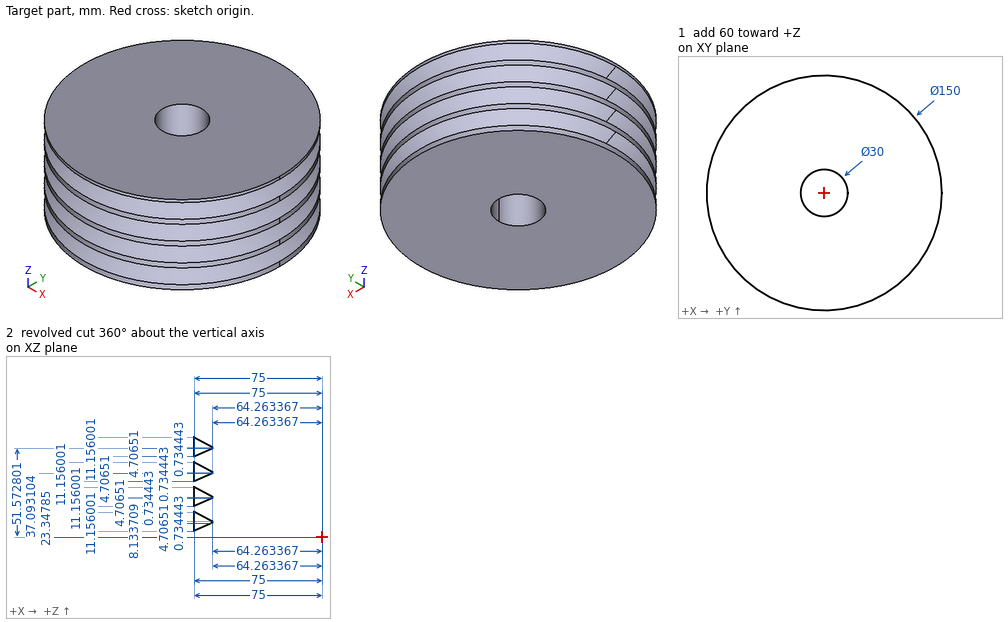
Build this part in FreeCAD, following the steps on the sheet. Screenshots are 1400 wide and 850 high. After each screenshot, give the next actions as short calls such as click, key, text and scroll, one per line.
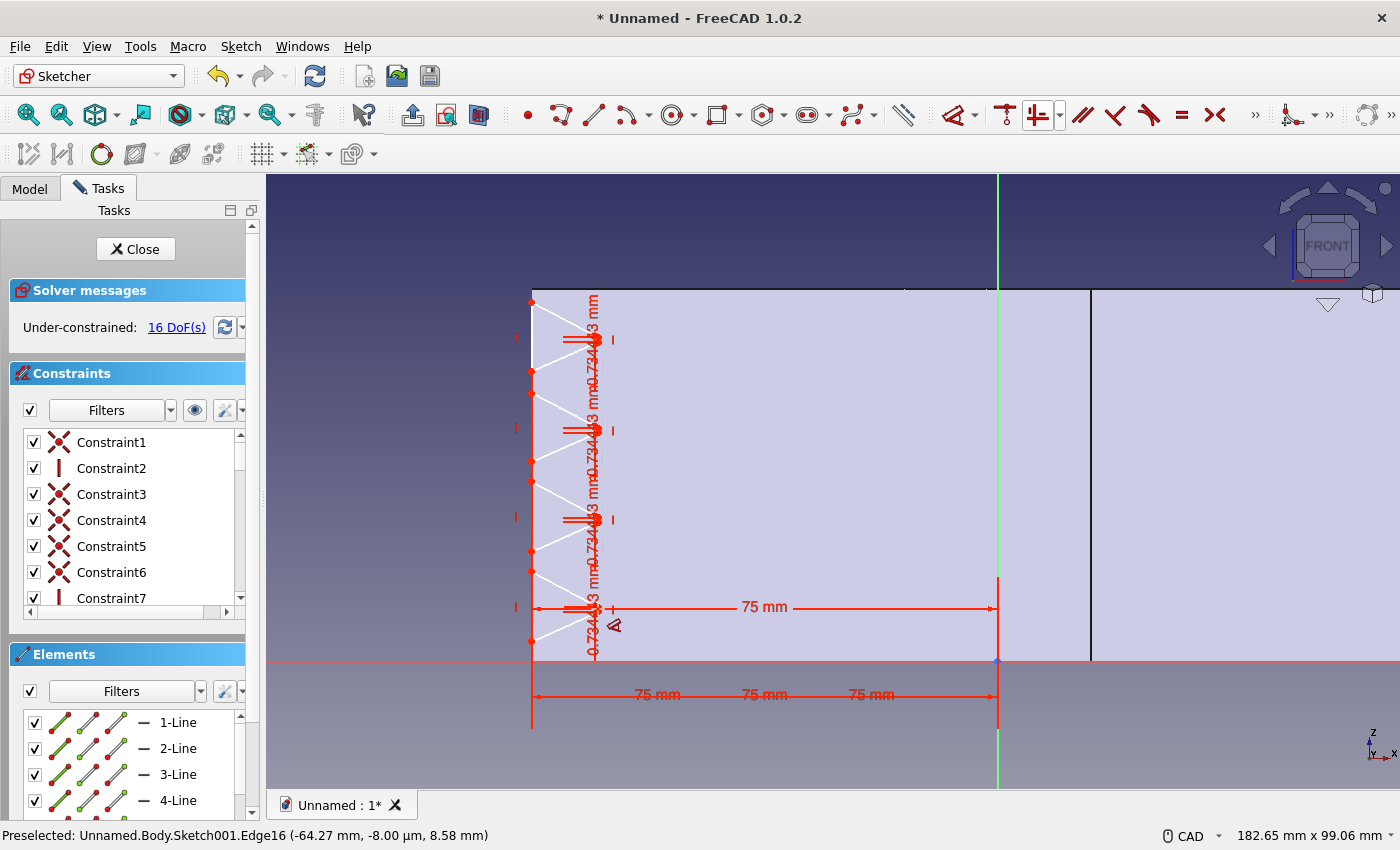
scroll(578, 351, up, 2)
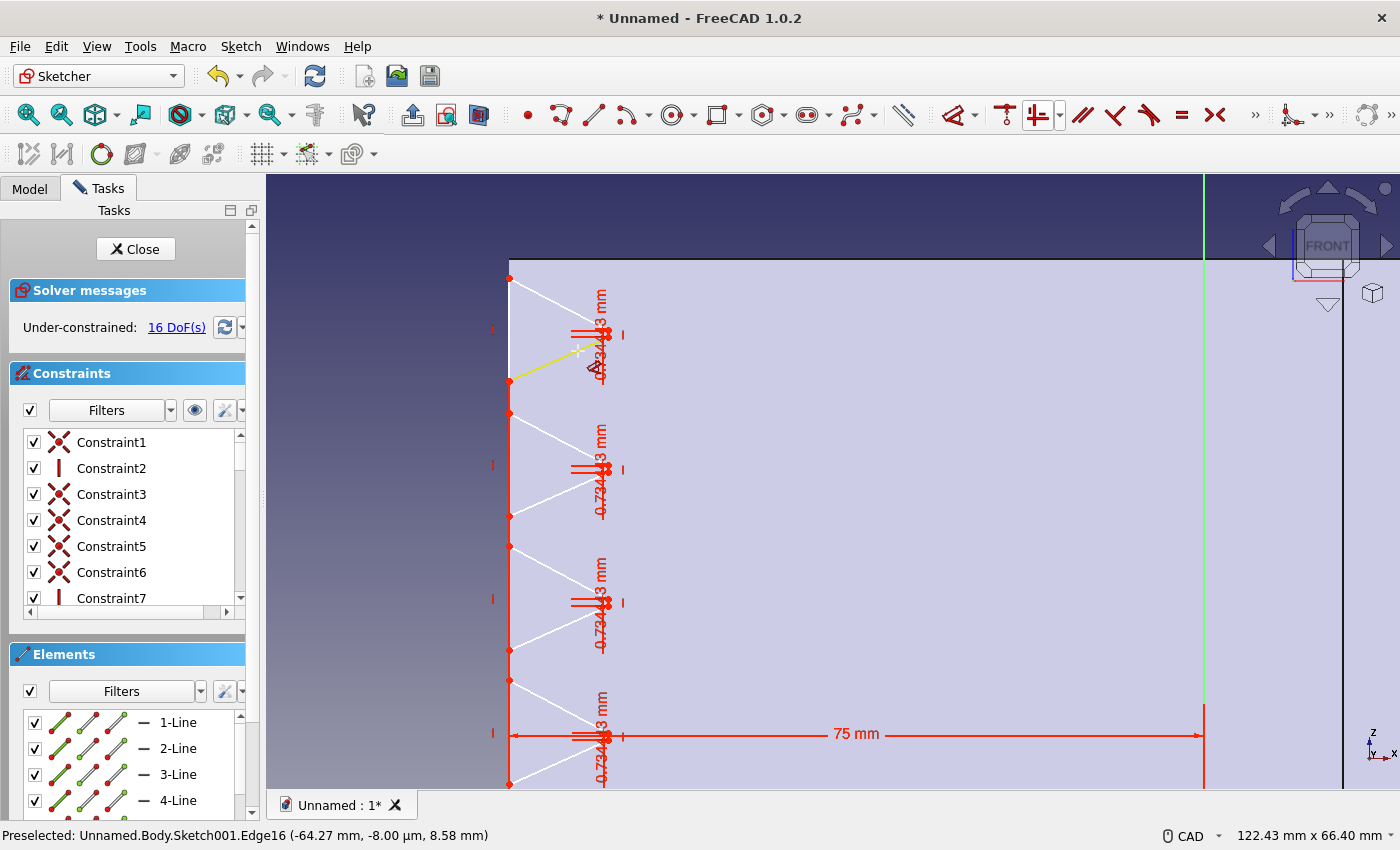
click(579, 351)
click(475, 359)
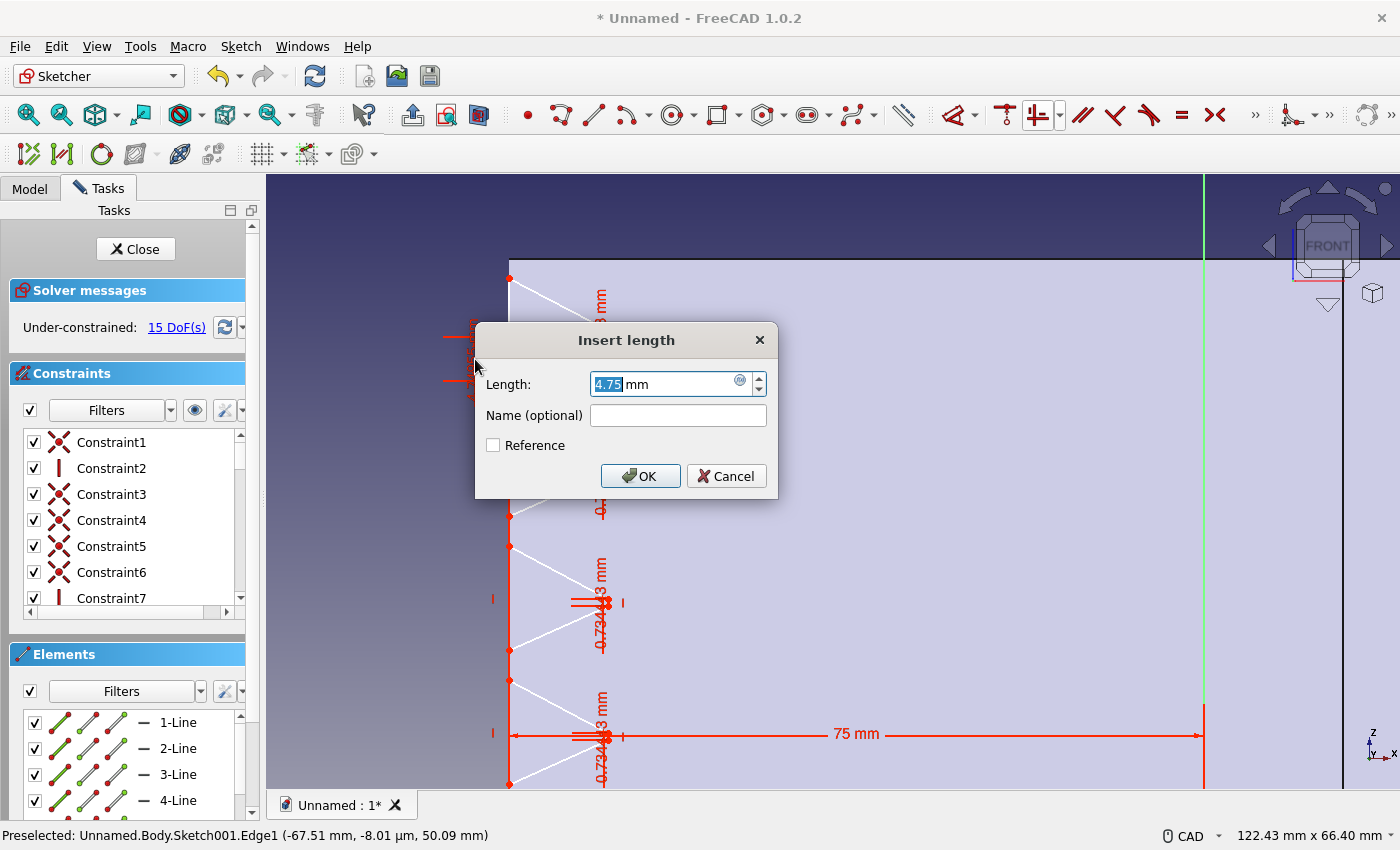
text(4.70651)
key(Return)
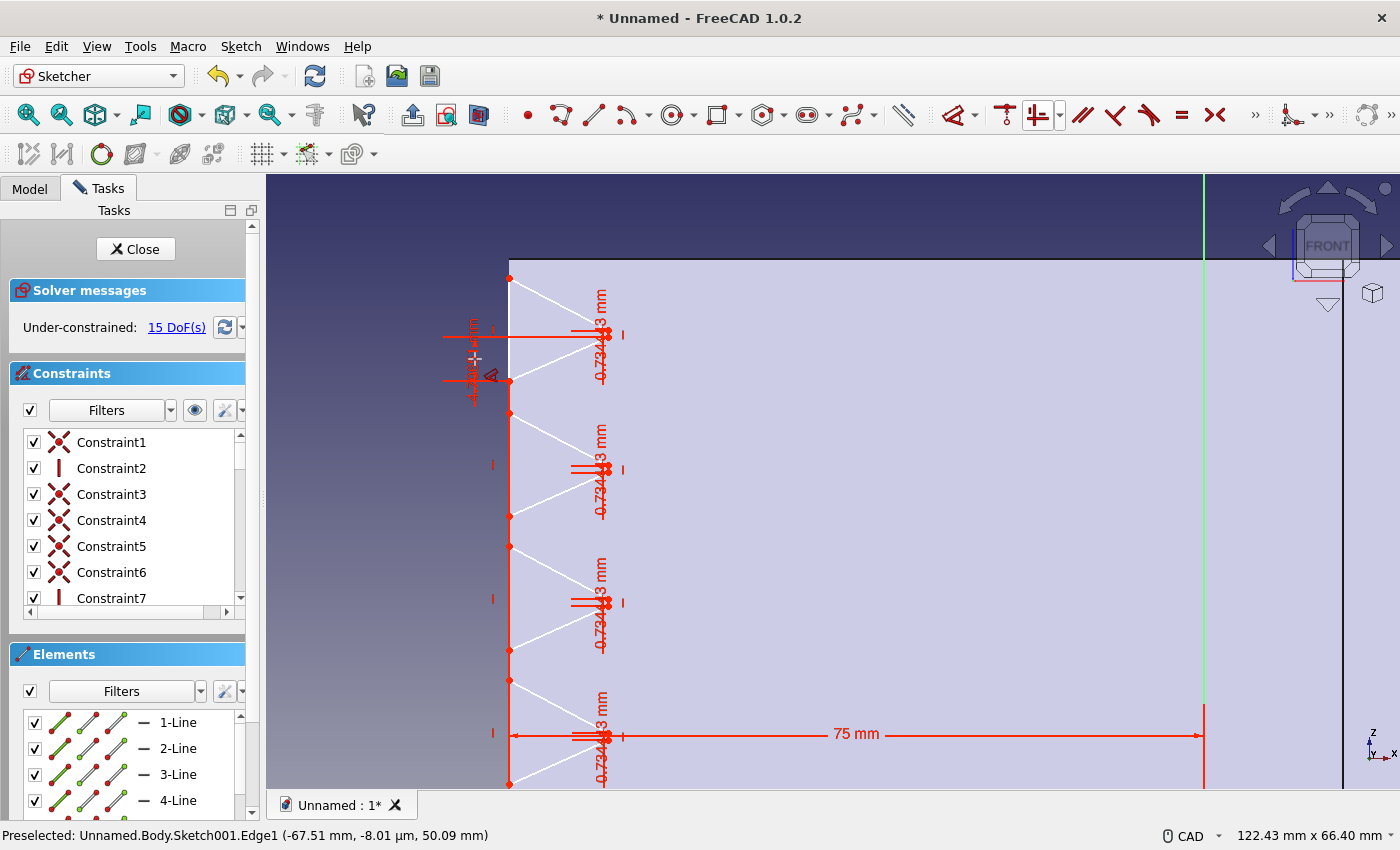
click(579, 486)
click(475, 494)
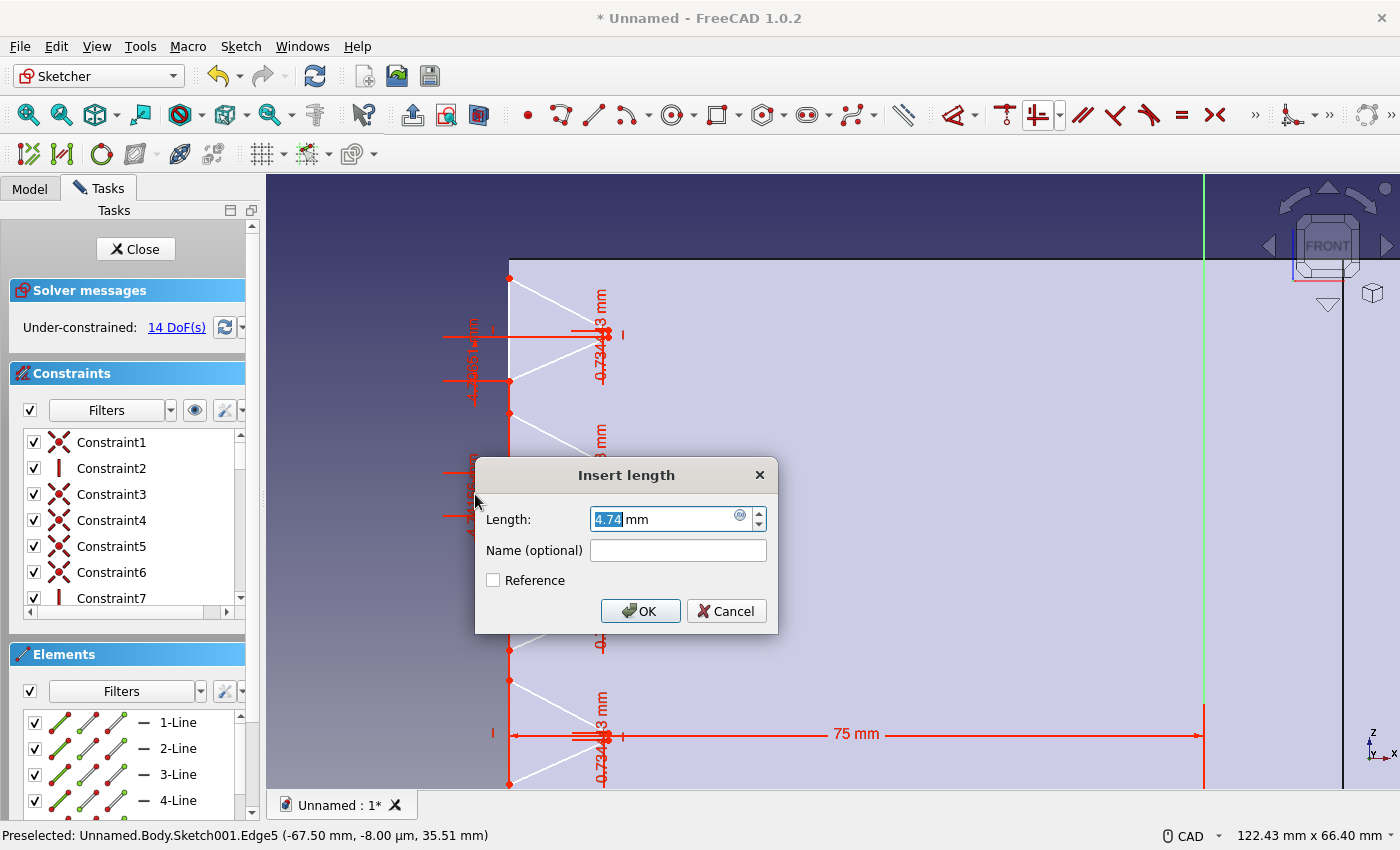
text(4.70651)
key(Return)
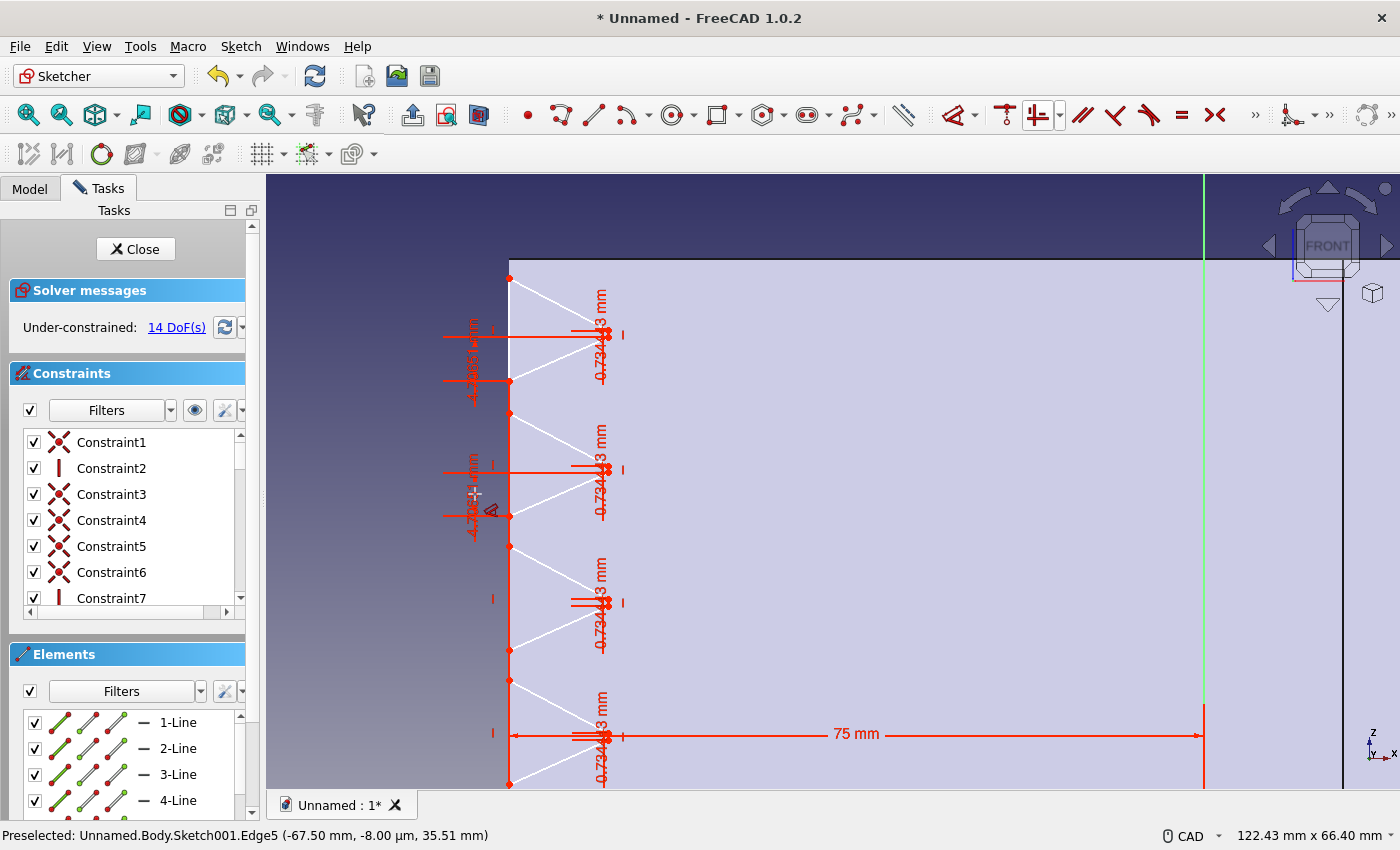
click(579, 620)
click(475, 628)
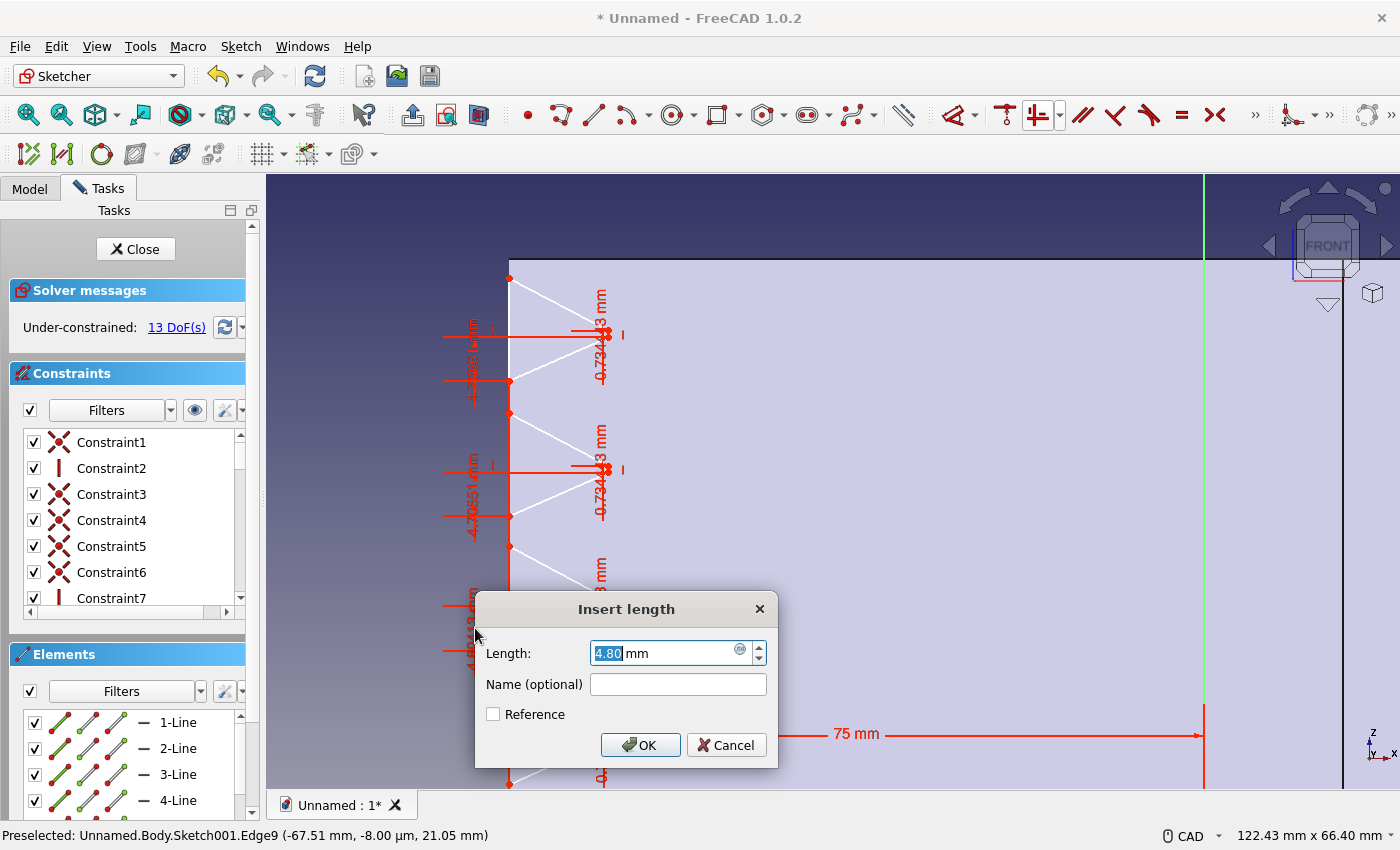
text(4.70651)
key(Return)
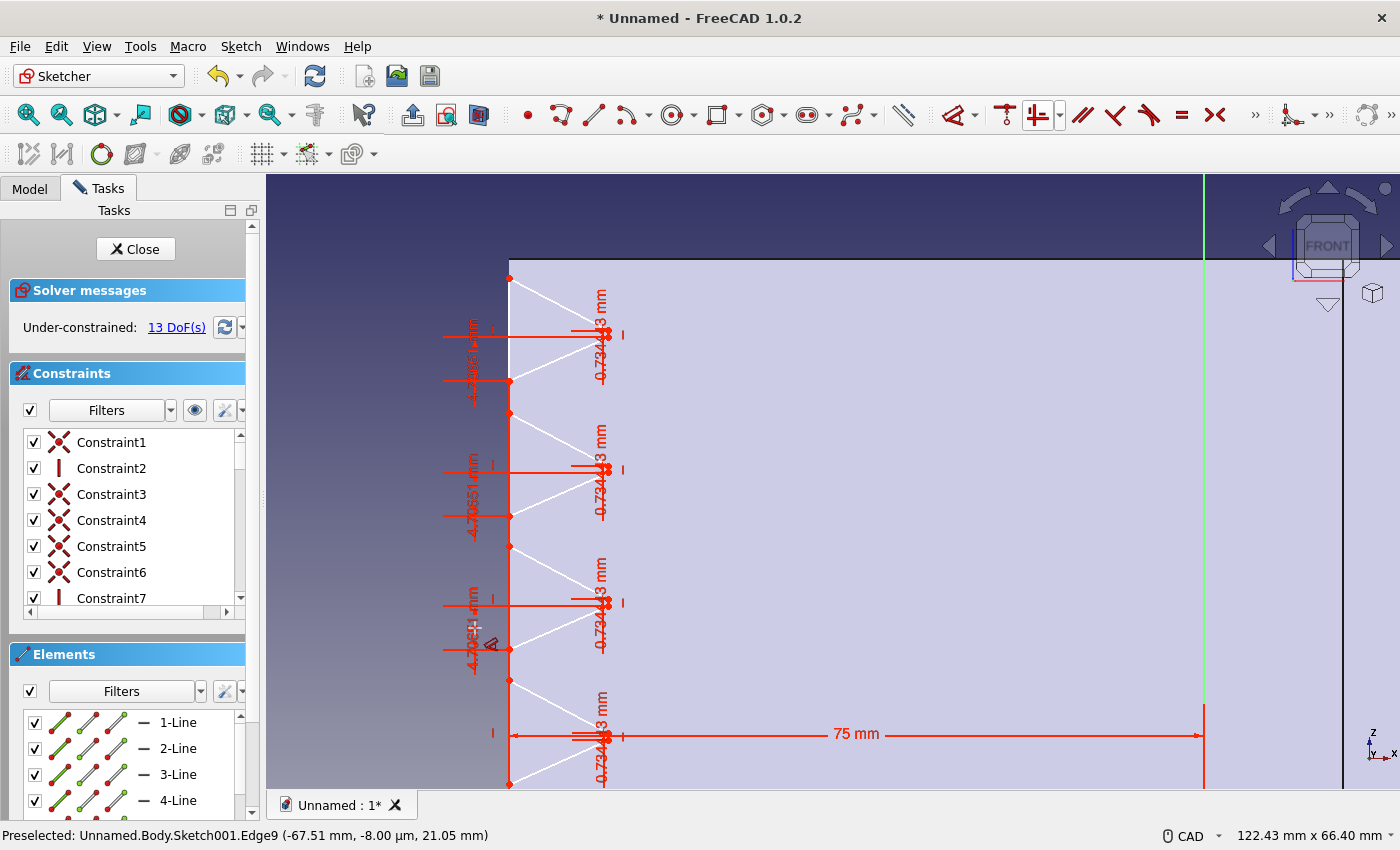
click(579, 754)
click(475, 751)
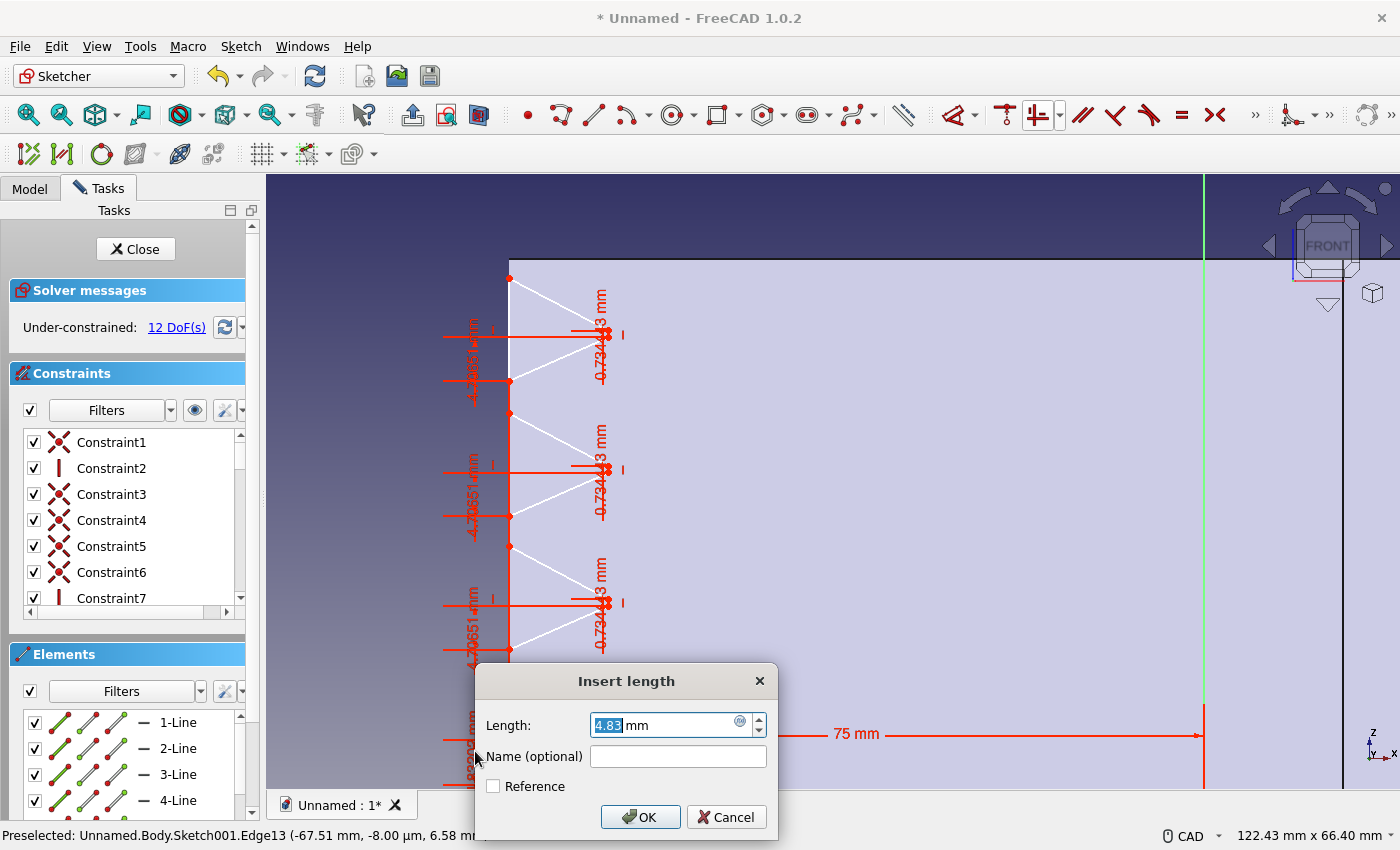
text(4.70651)
key(Return)